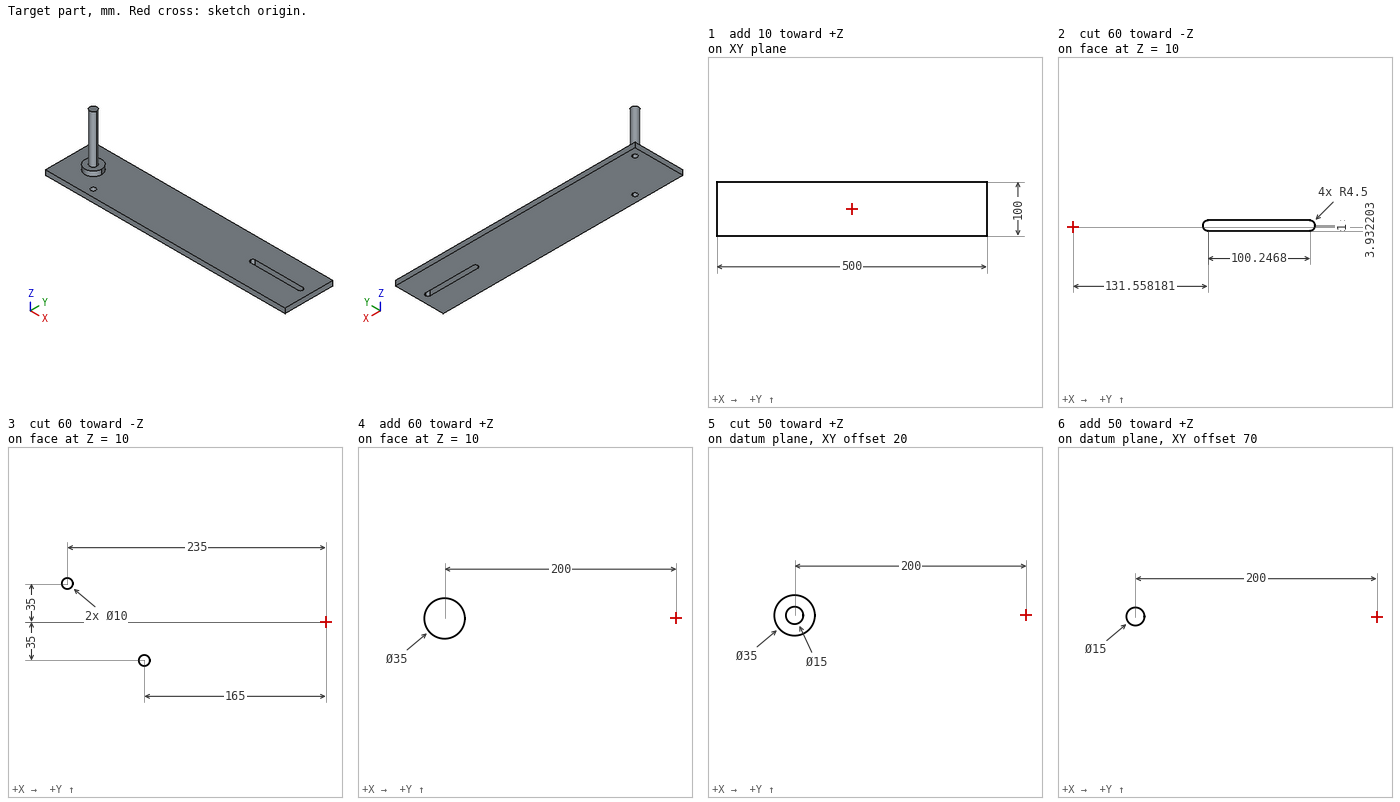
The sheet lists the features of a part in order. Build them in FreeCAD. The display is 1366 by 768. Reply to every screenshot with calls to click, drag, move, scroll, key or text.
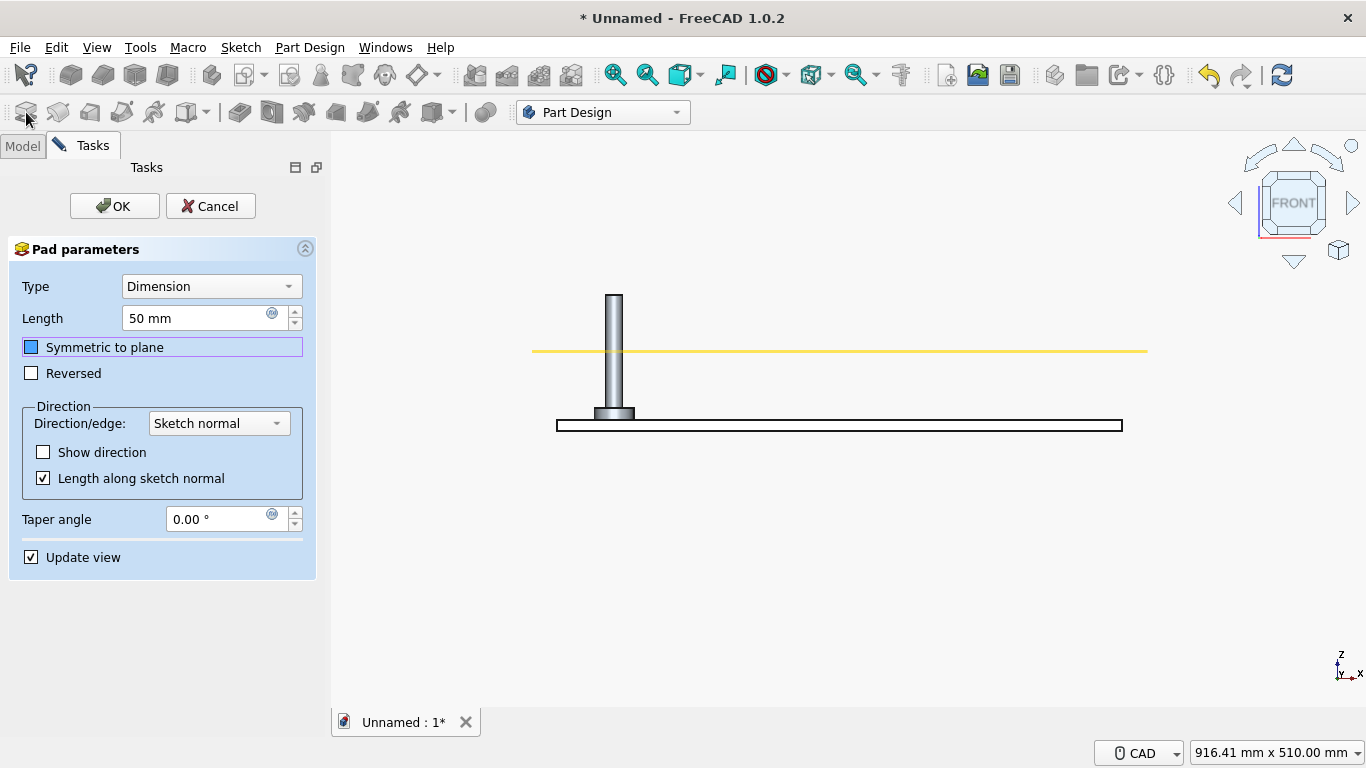
click(115, 206)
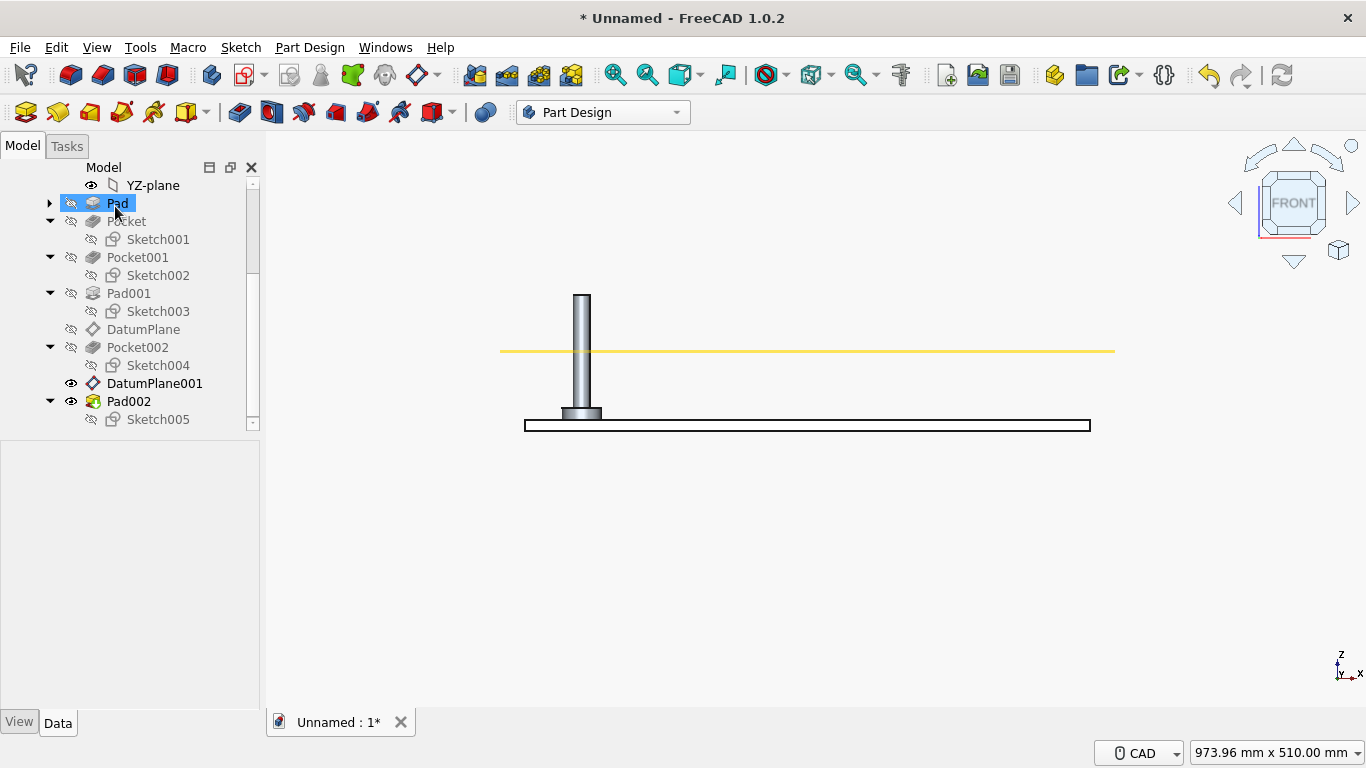
click(116, 383)
key(space)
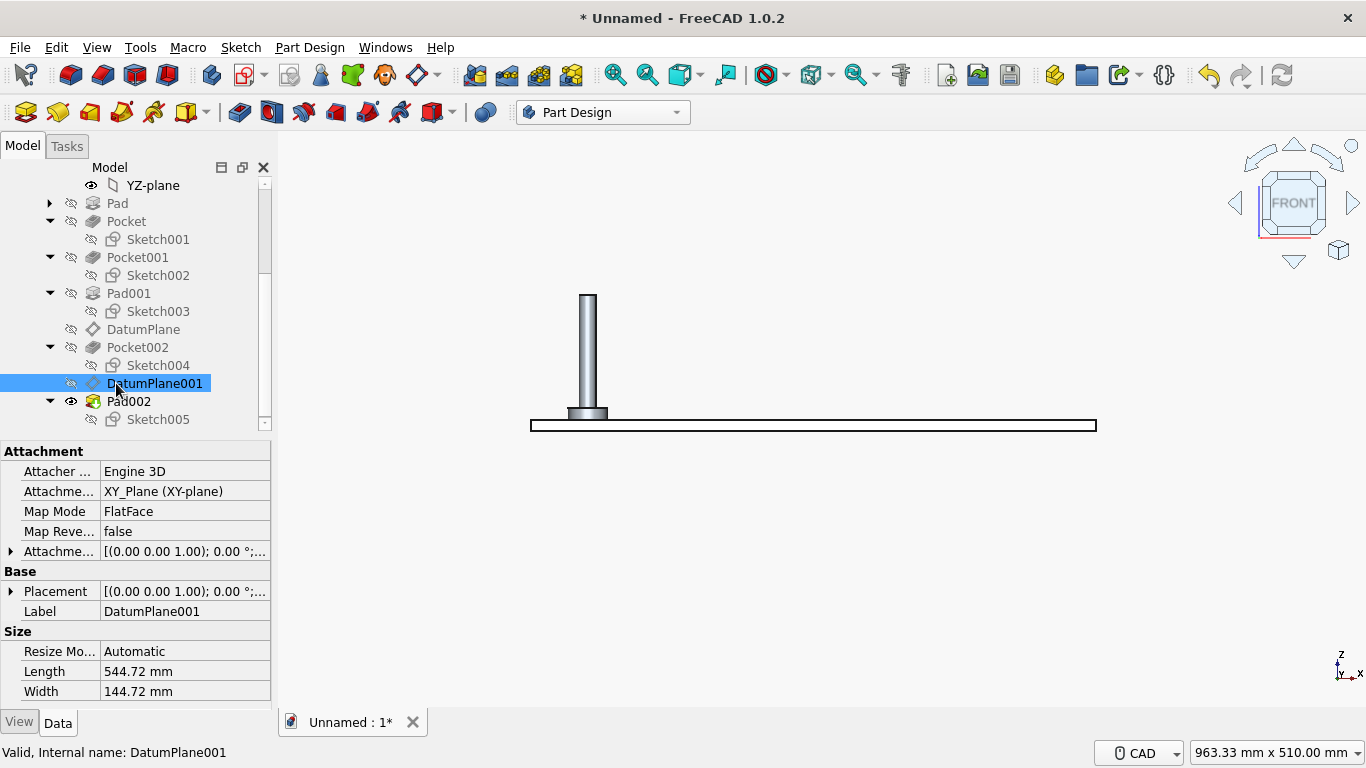
key(0)